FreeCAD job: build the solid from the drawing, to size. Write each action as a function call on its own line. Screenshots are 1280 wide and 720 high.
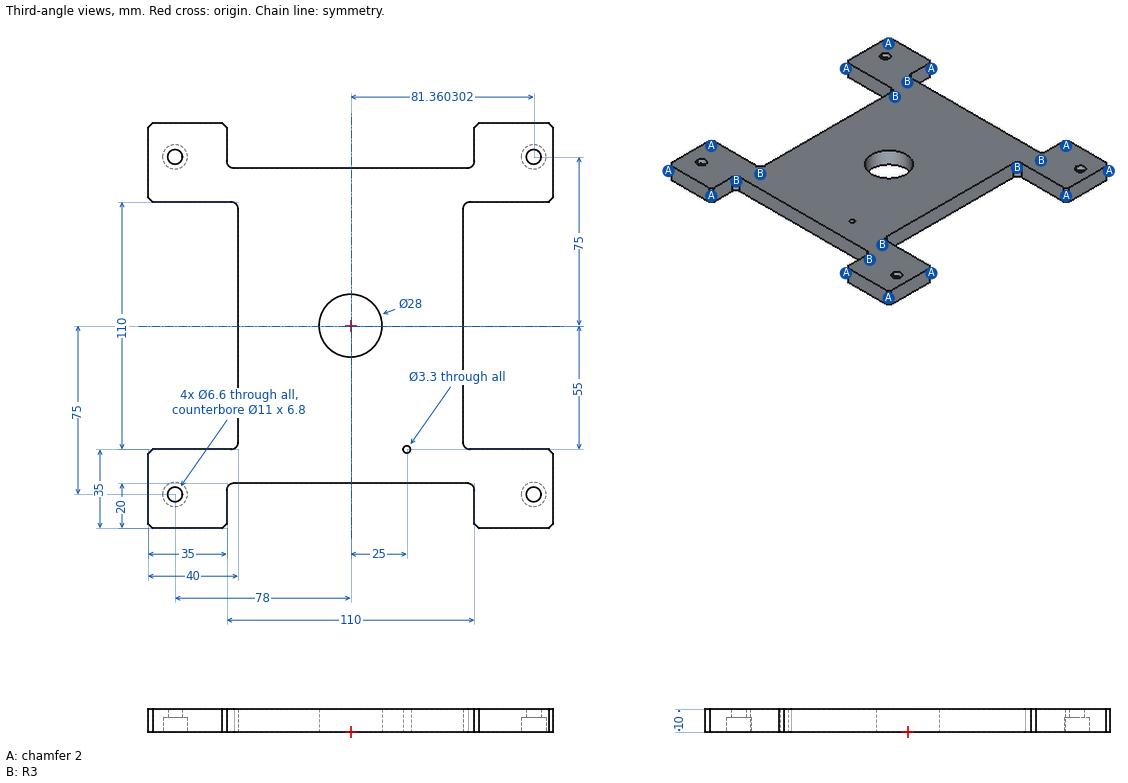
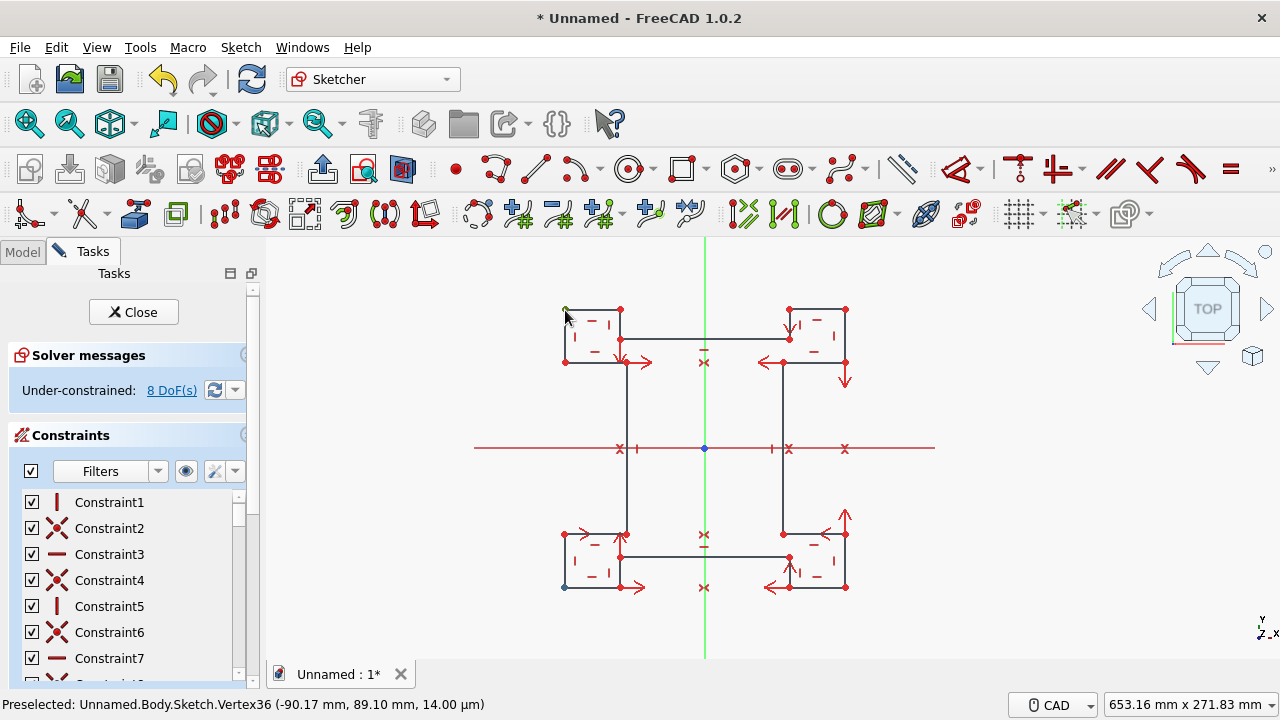
click(470, 448)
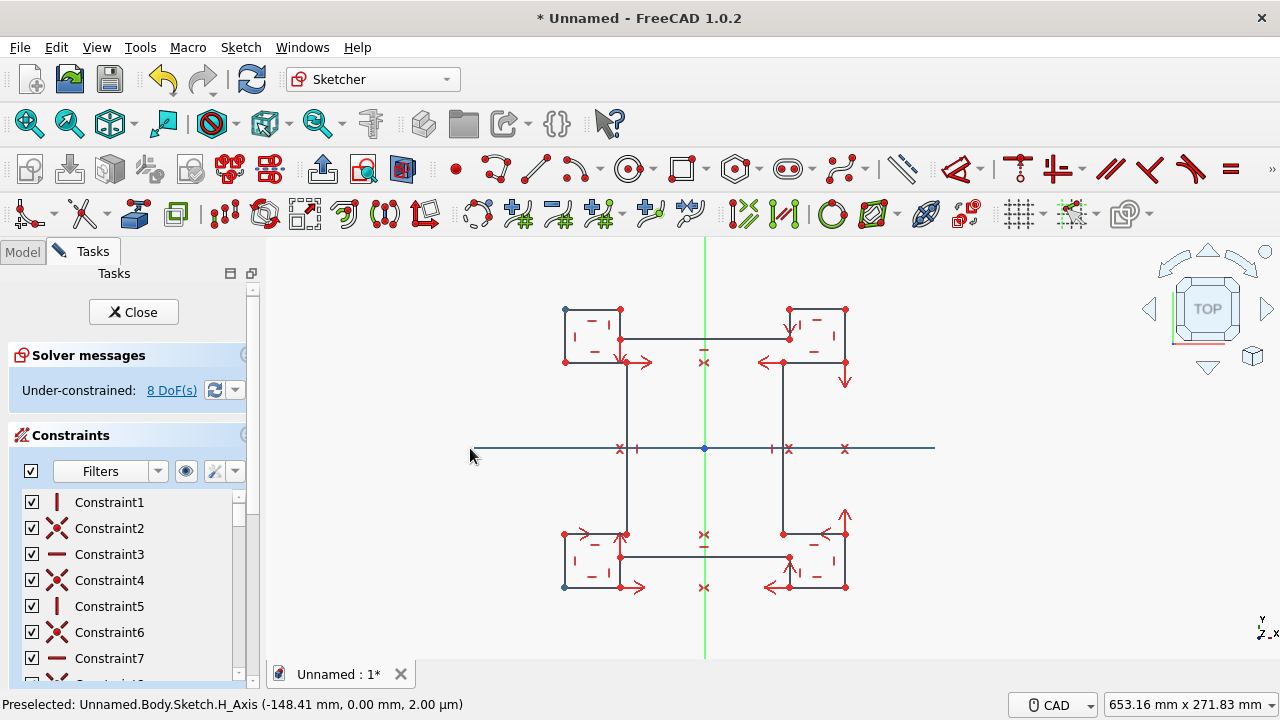
key(s)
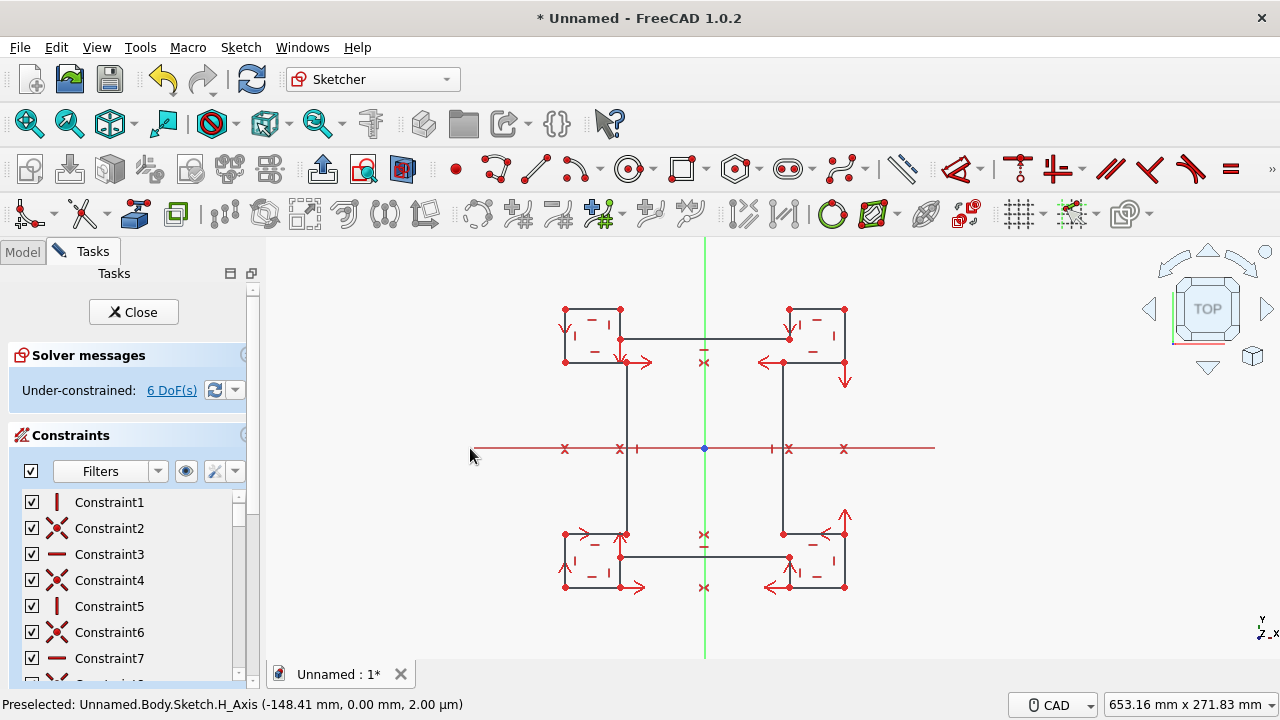
click(608, 534)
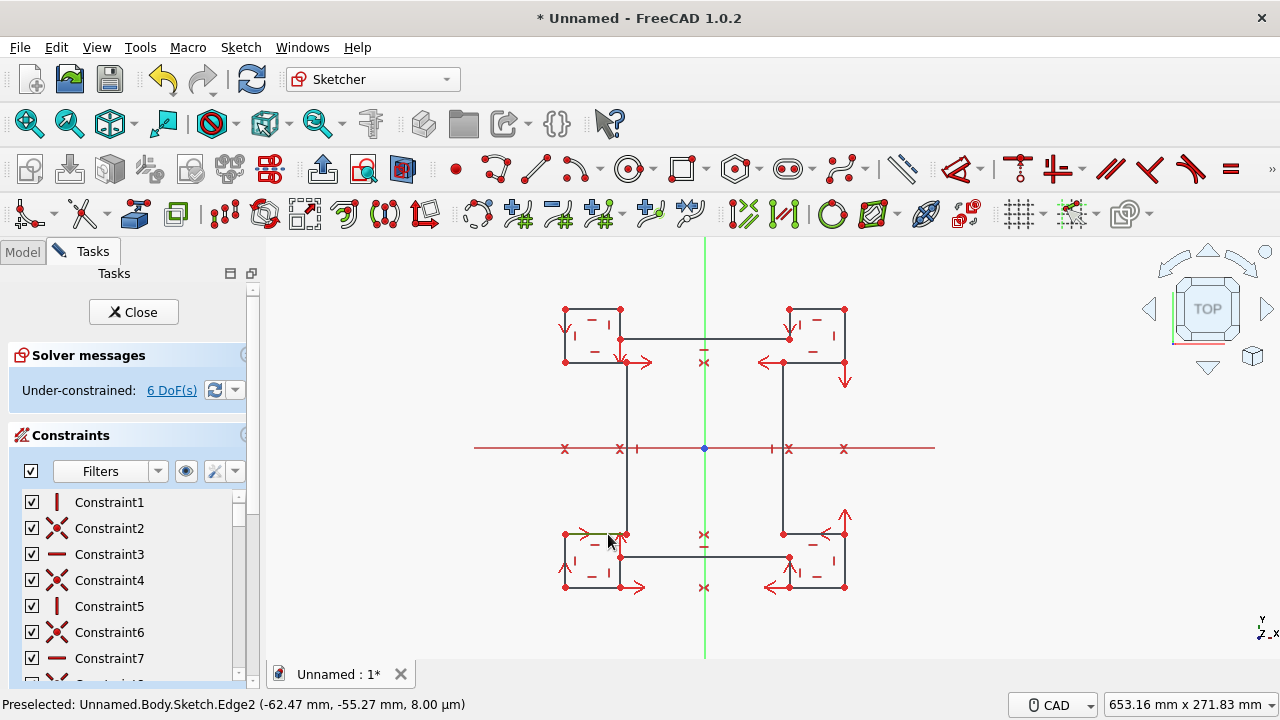
click(982, 170)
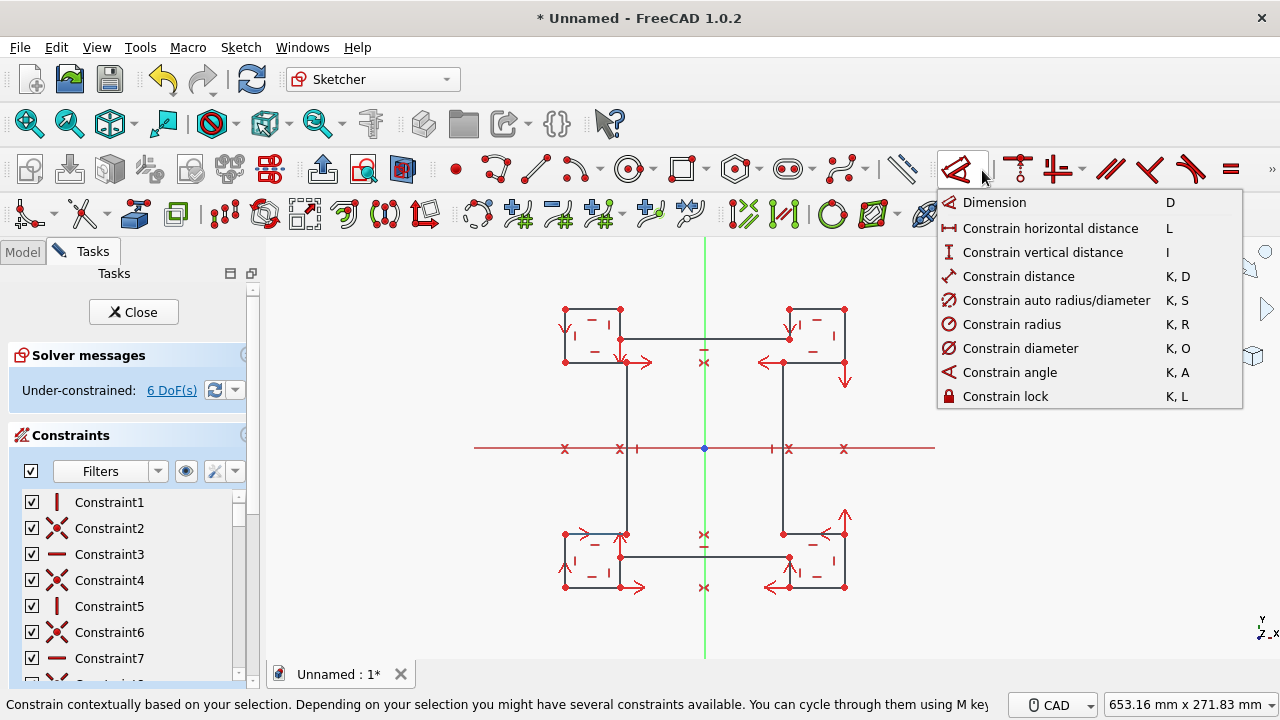
click(1090, 228)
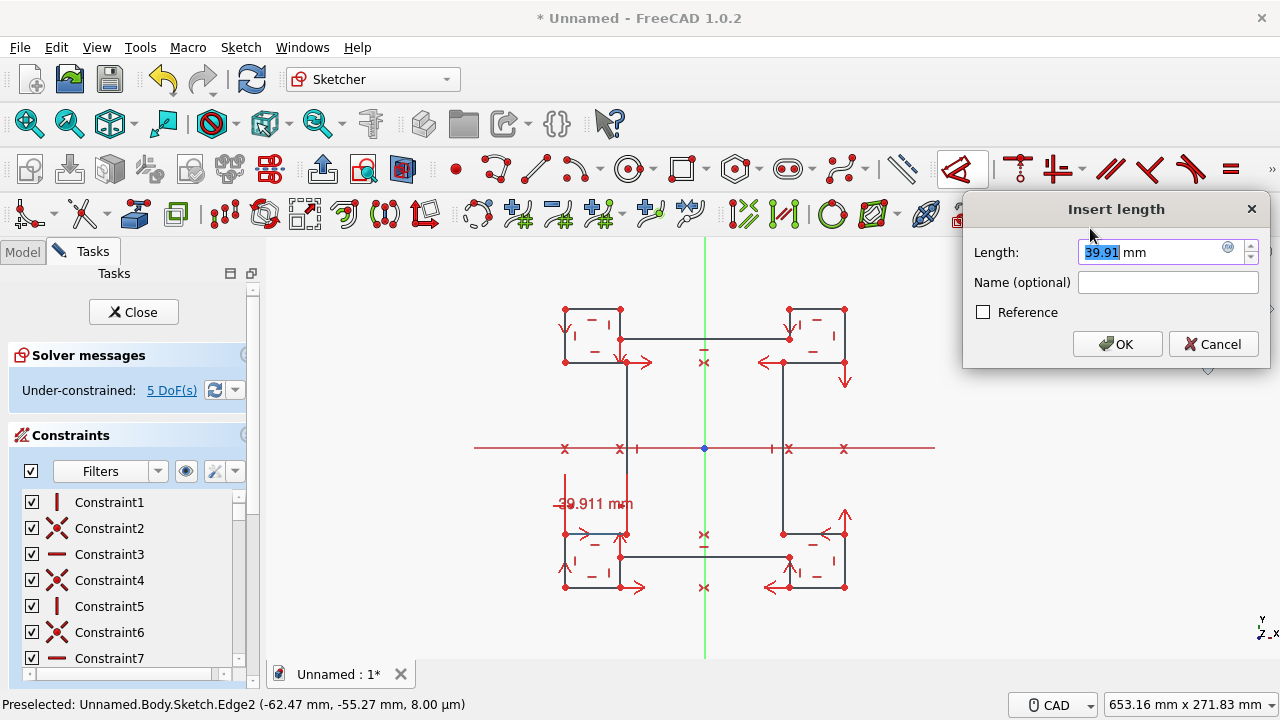
text(40)
key(Return)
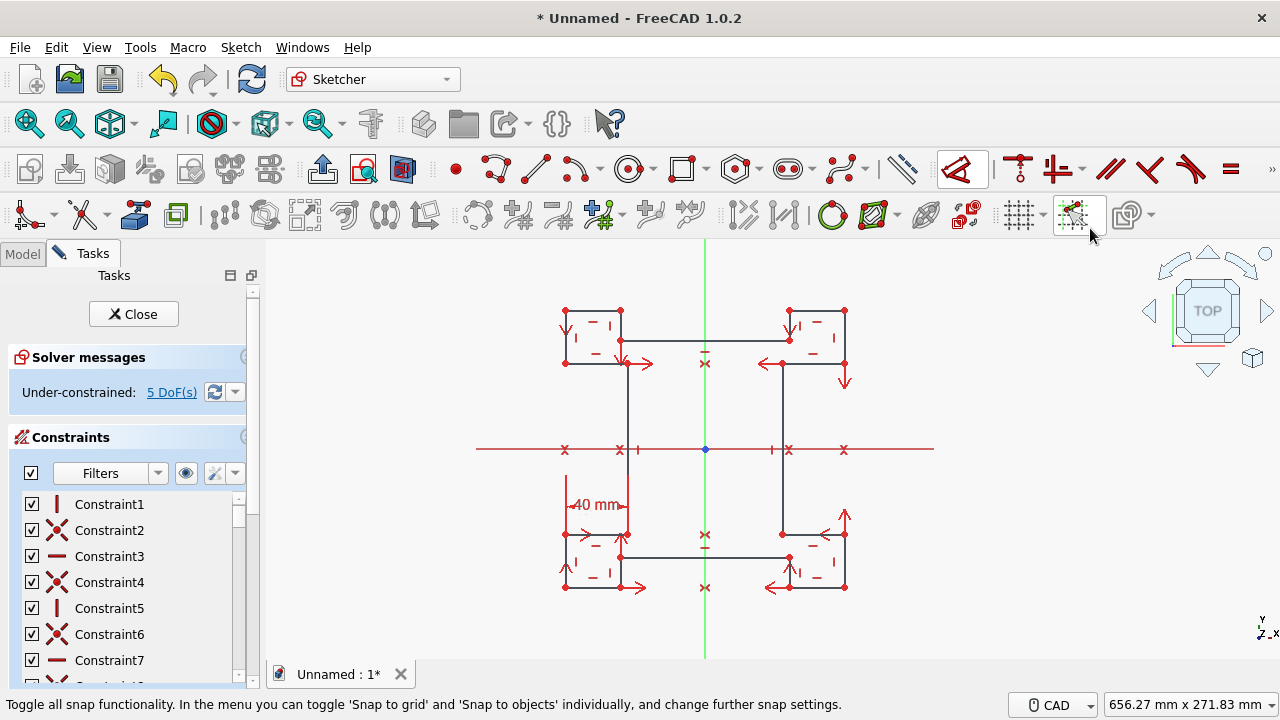
click(566, 551)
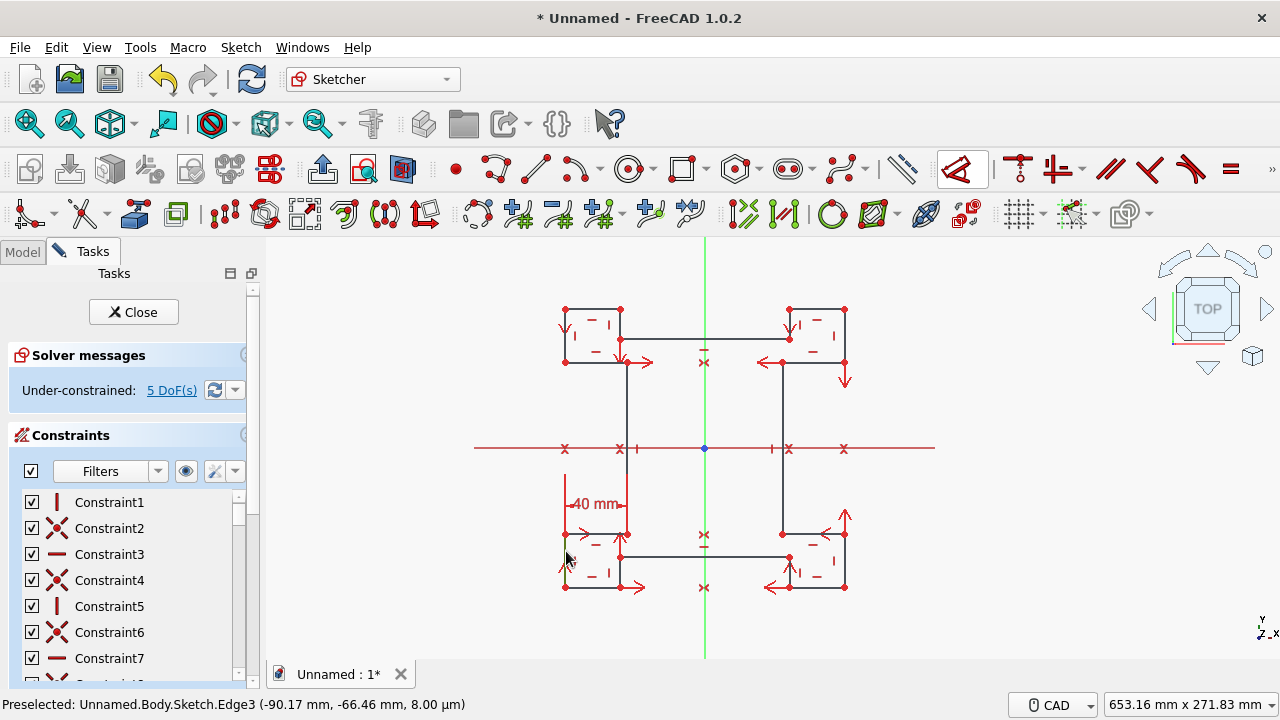
click(982, 170)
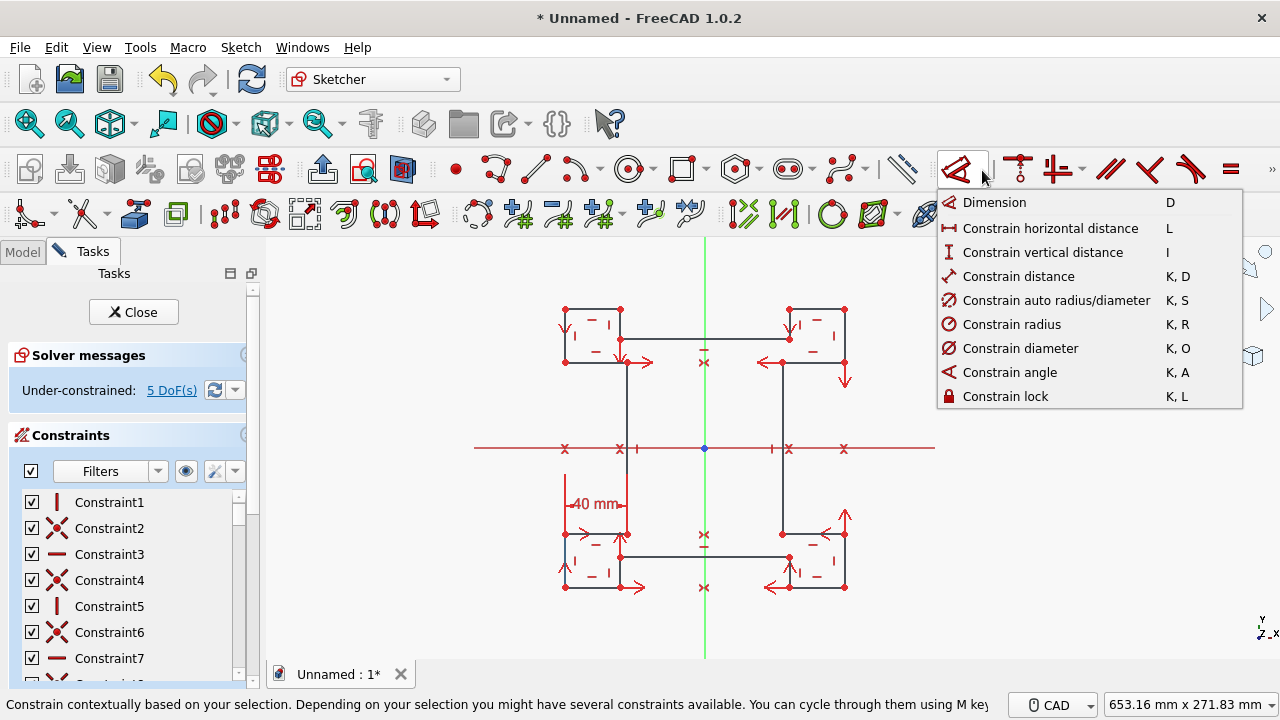
click(1090, 252)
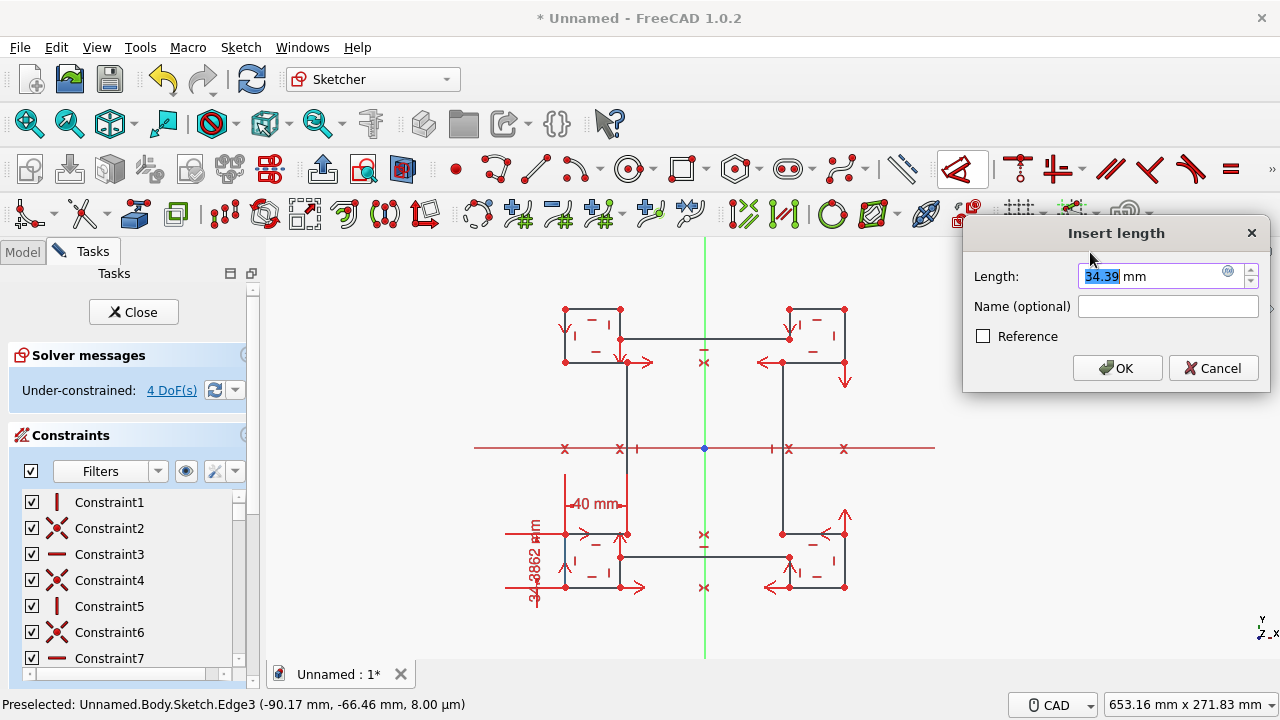
text(35)
key(Return)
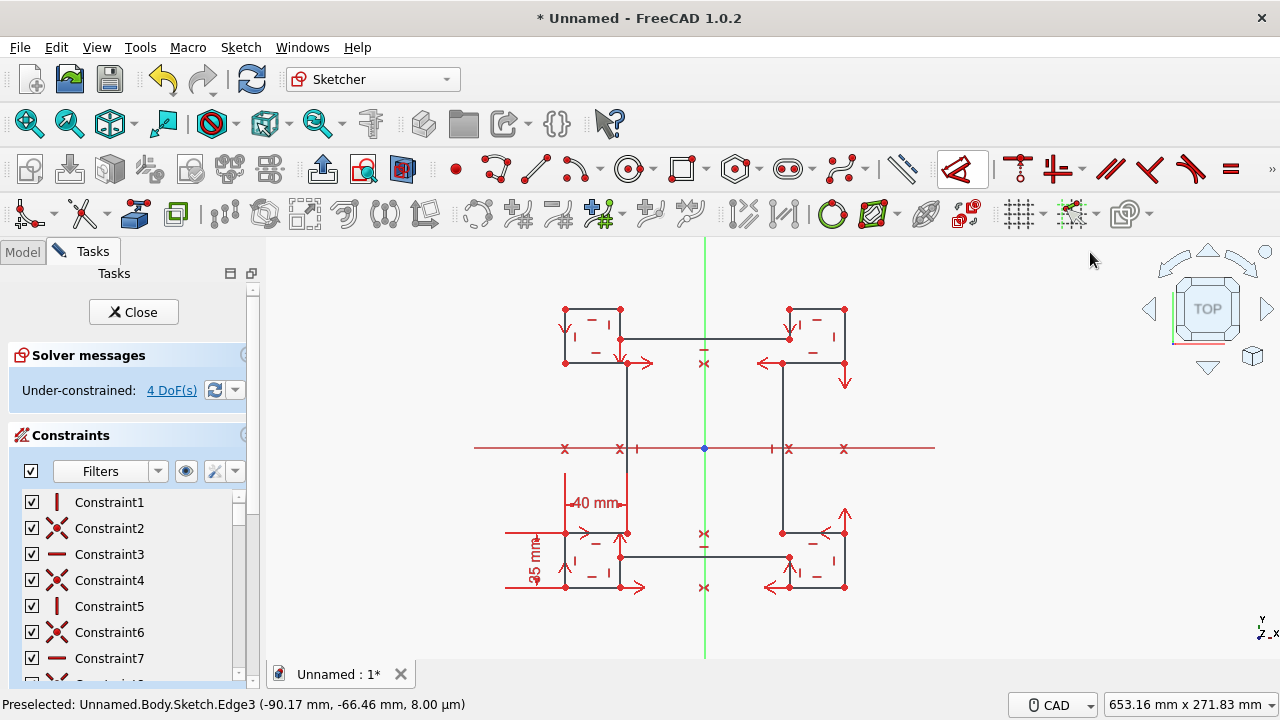
click(582, 588)